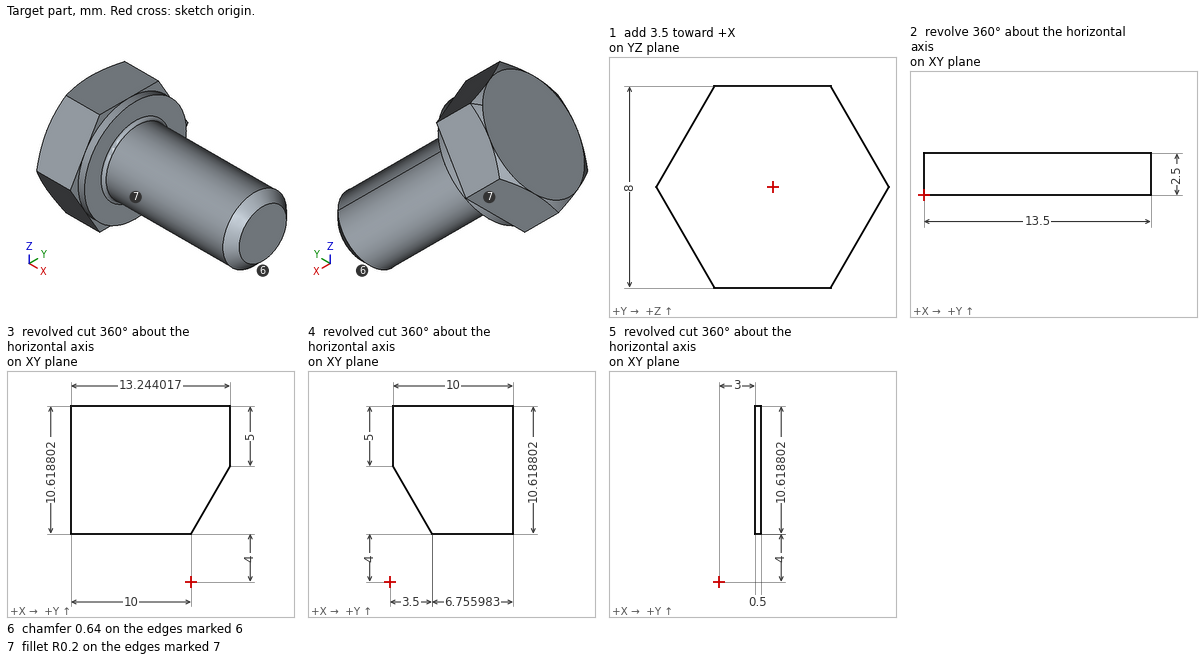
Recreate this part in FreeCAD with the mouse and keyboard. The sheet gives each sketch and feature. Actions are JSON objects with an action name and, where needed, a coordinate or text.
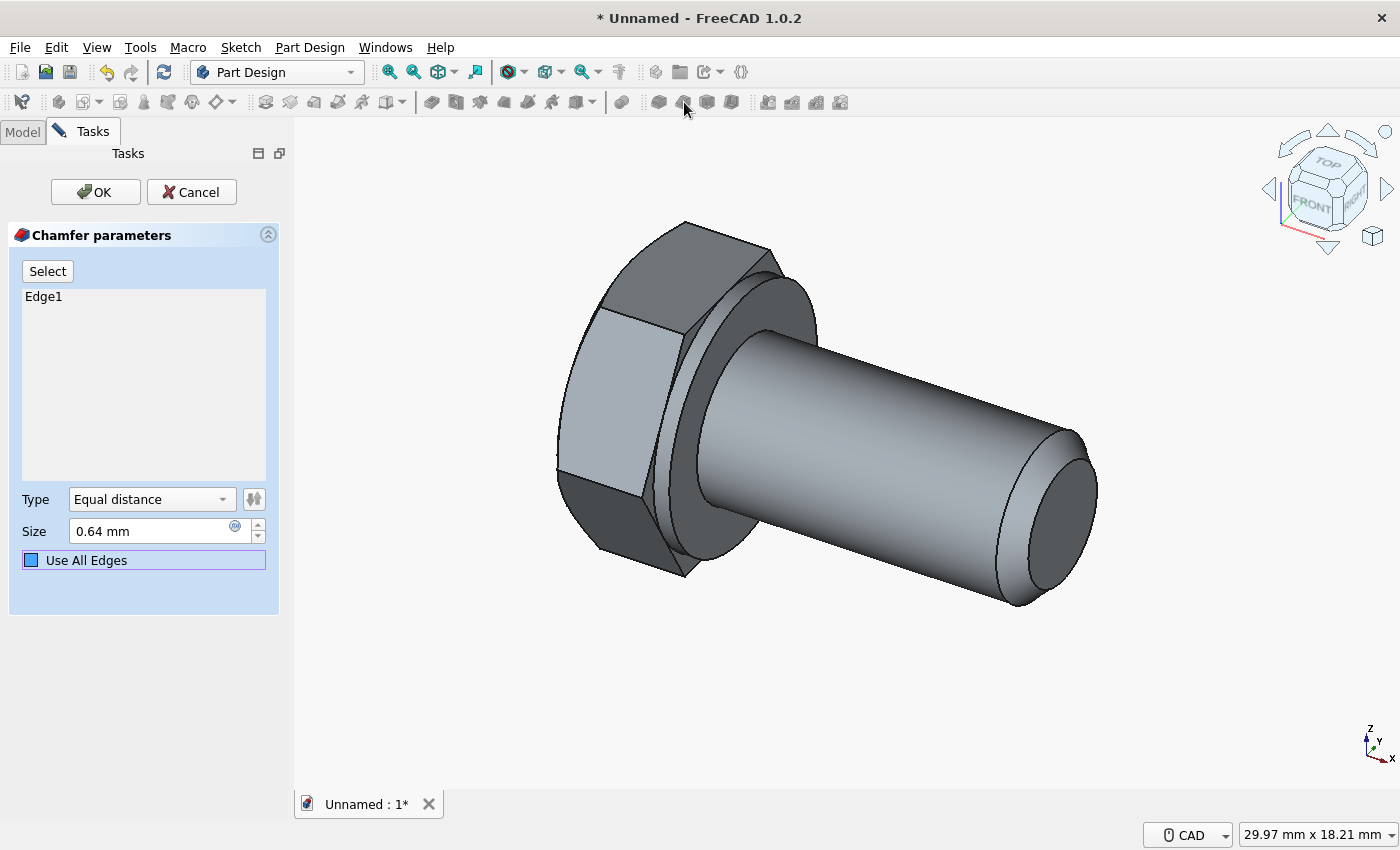
{"action": "left_click", "coordinate": [96, 192]}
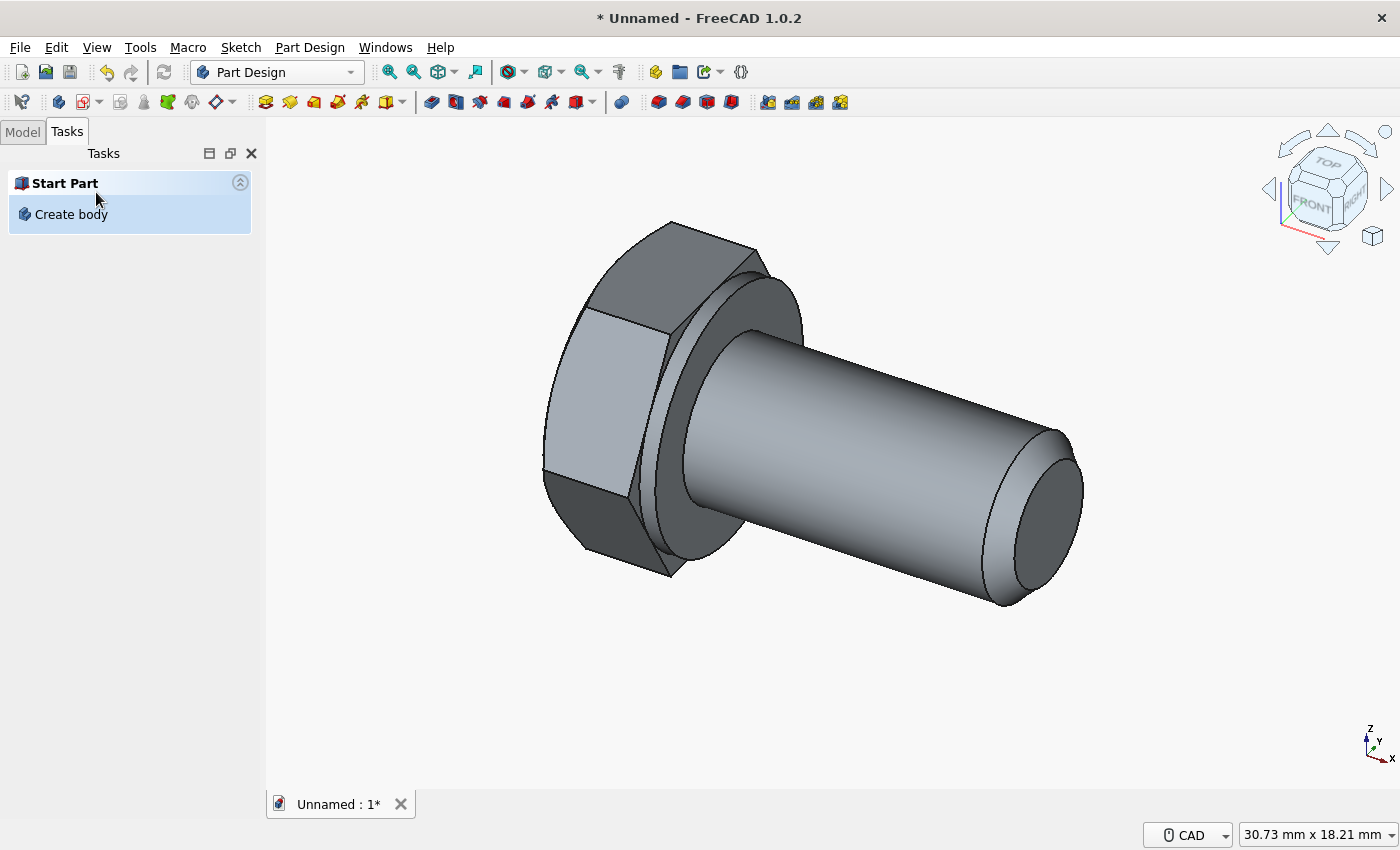
{"action": "key", "text": "0"}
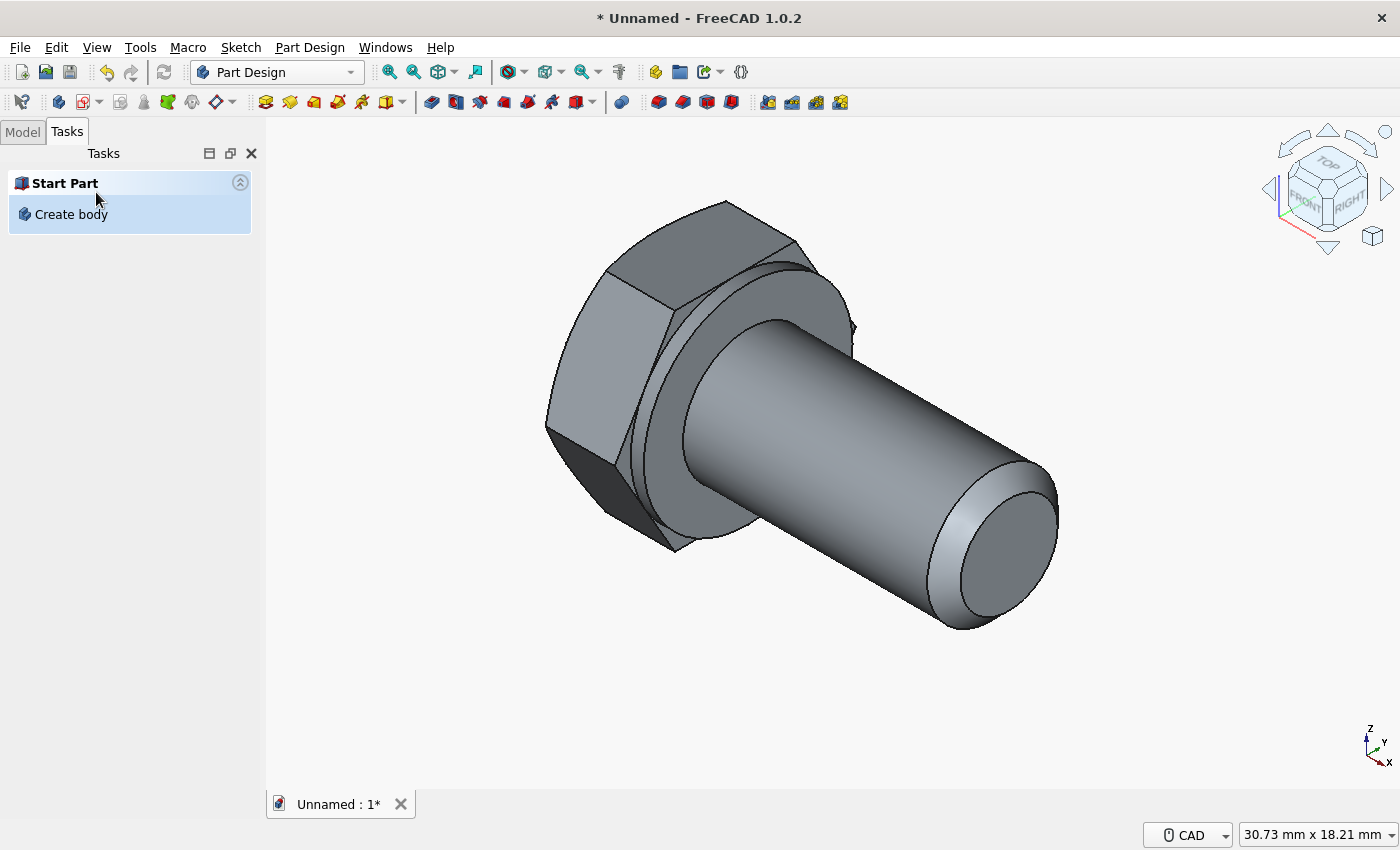
{"action": "key", "text": "2"}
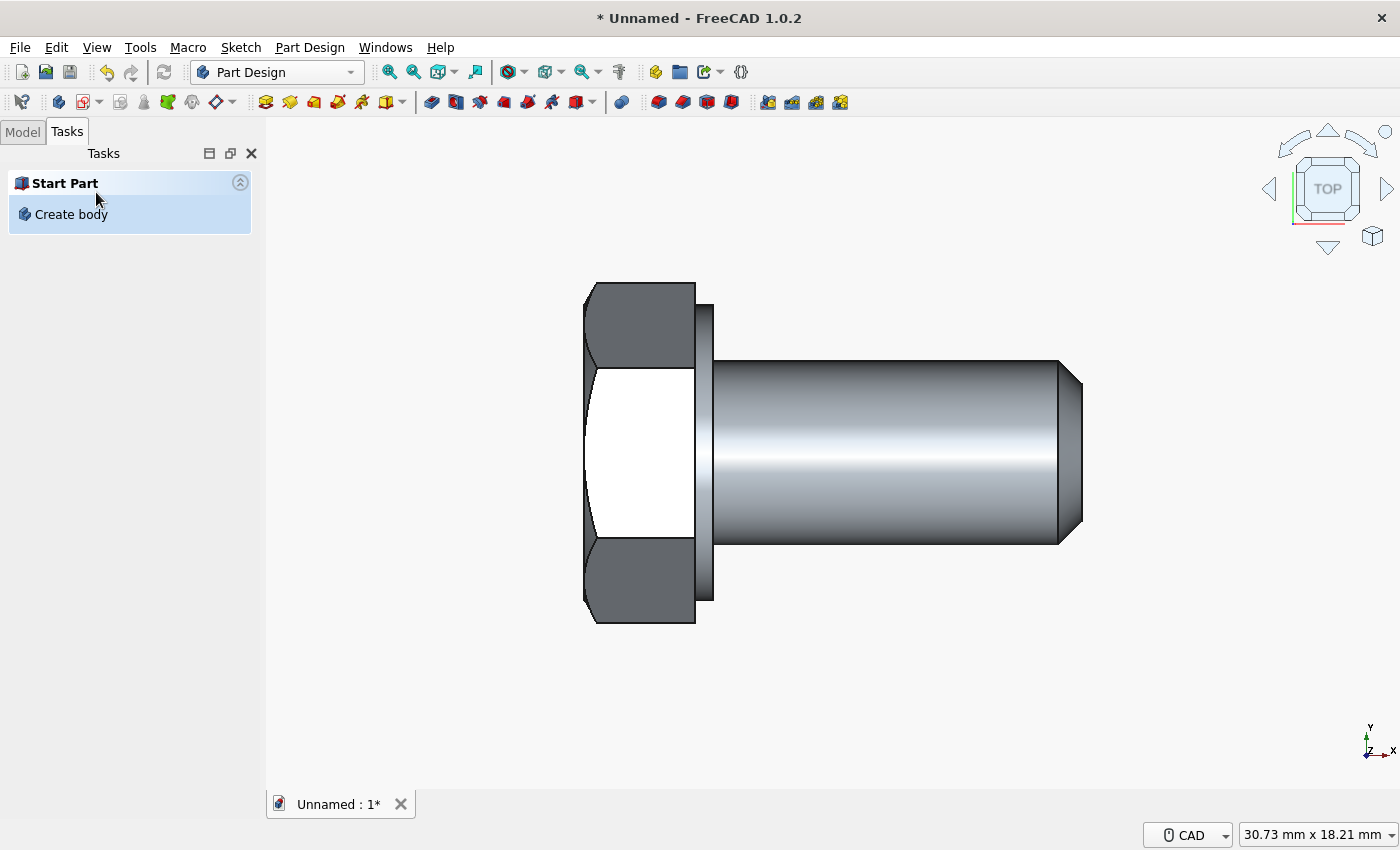
{"action": "key", "text": "1"}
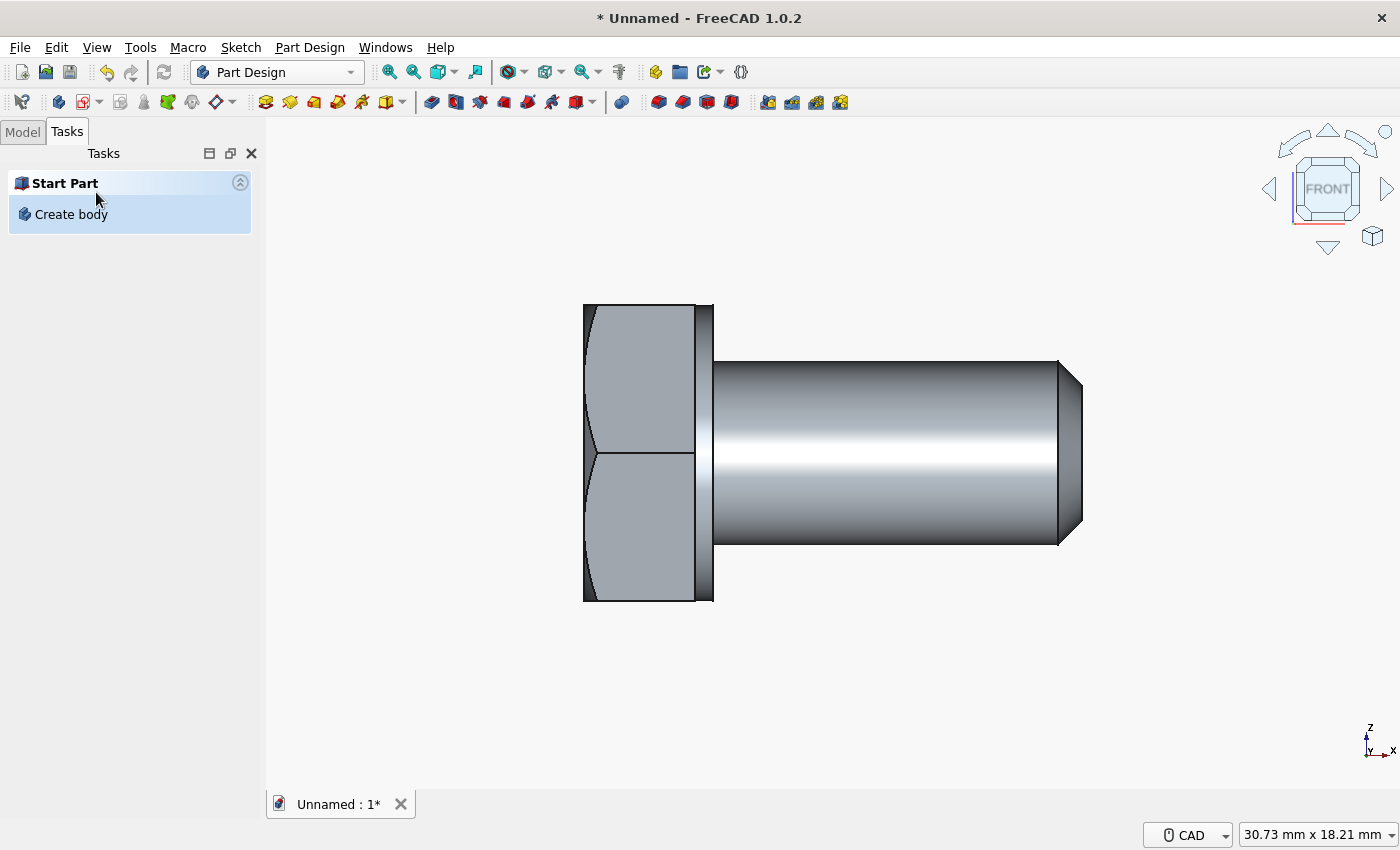
{"action": "left_click", "coordinate": [390, 72]}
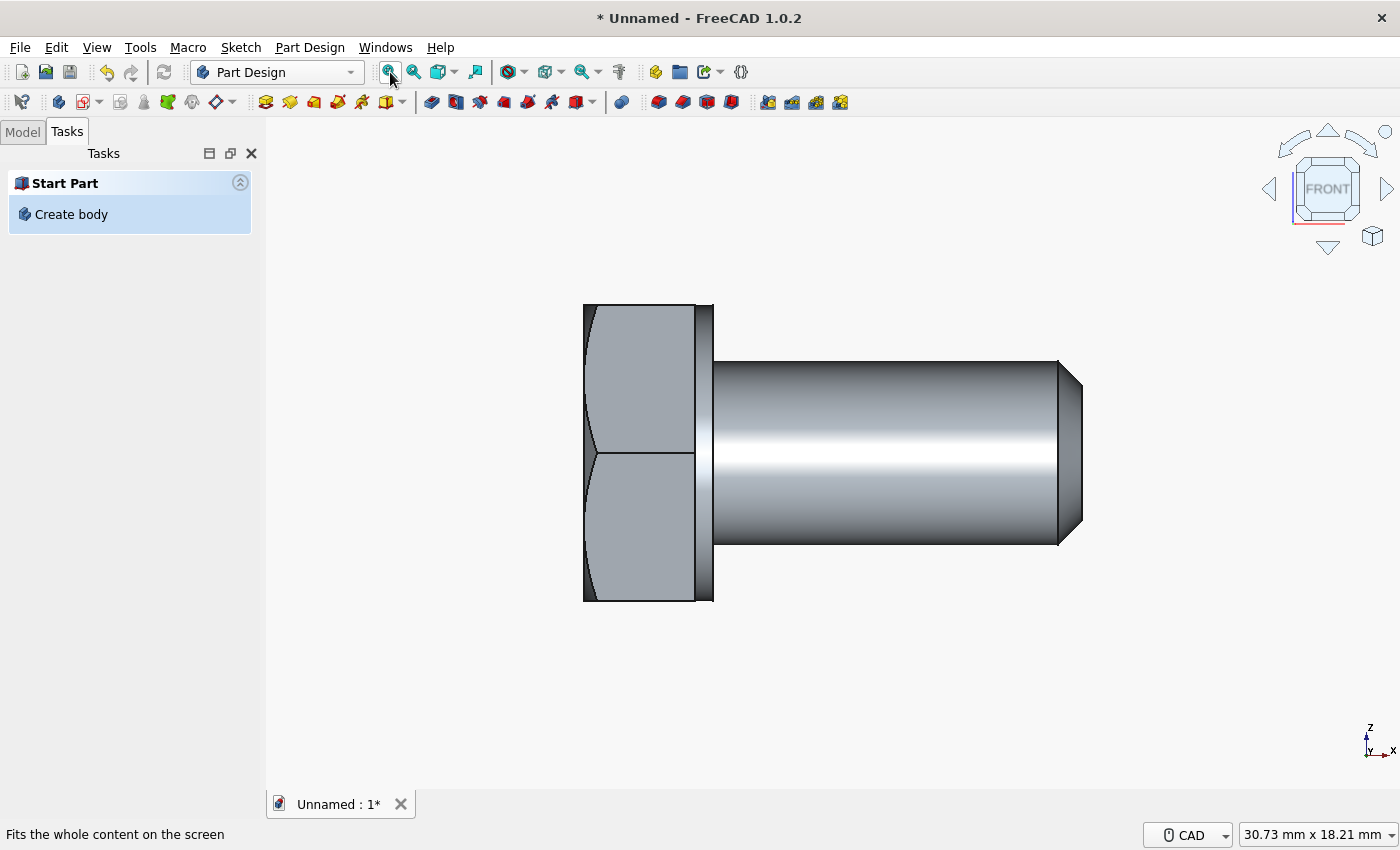
{"action": "key", "text": "3"}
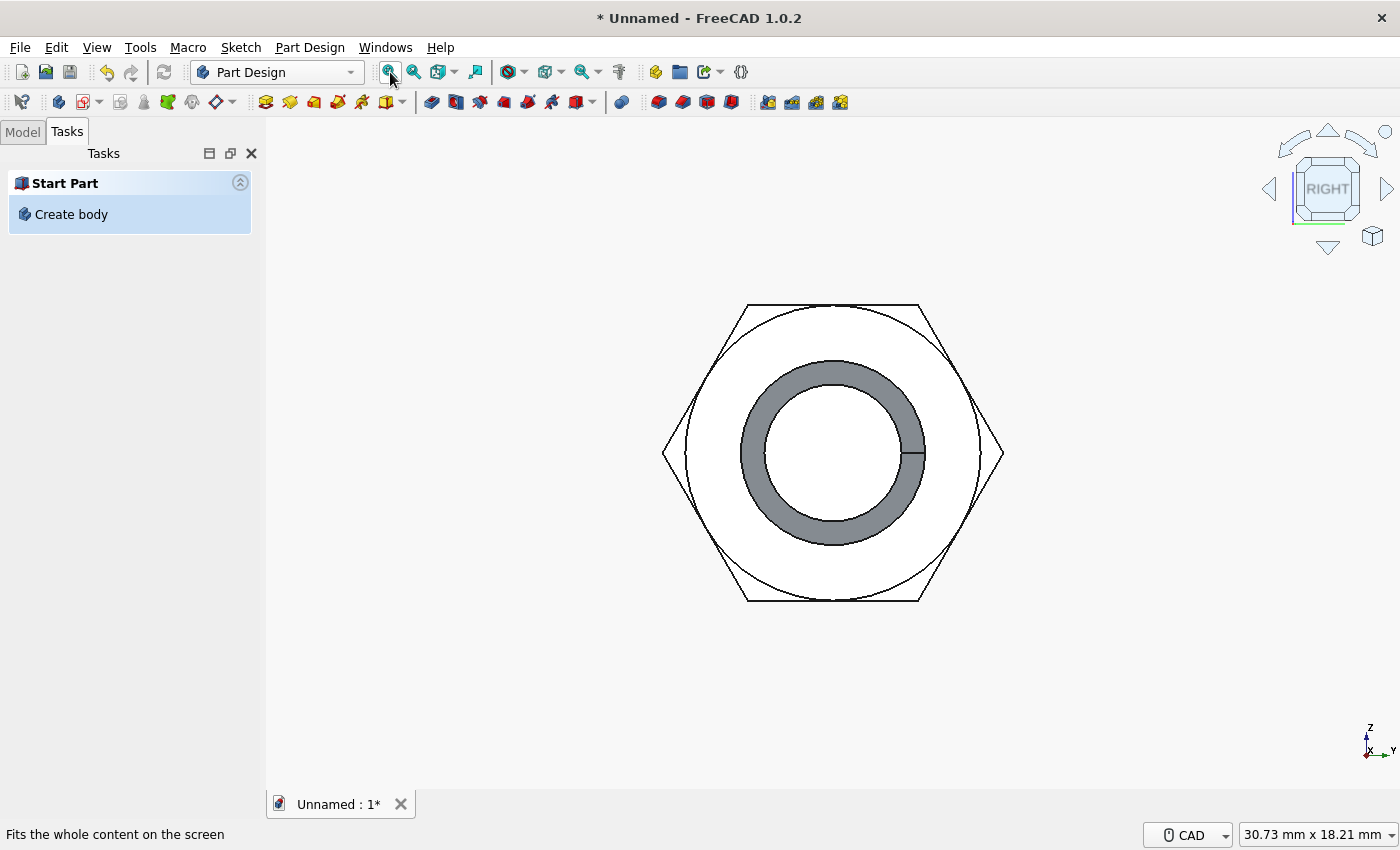
{"action": "left_click", "coordinate": [390, 72]}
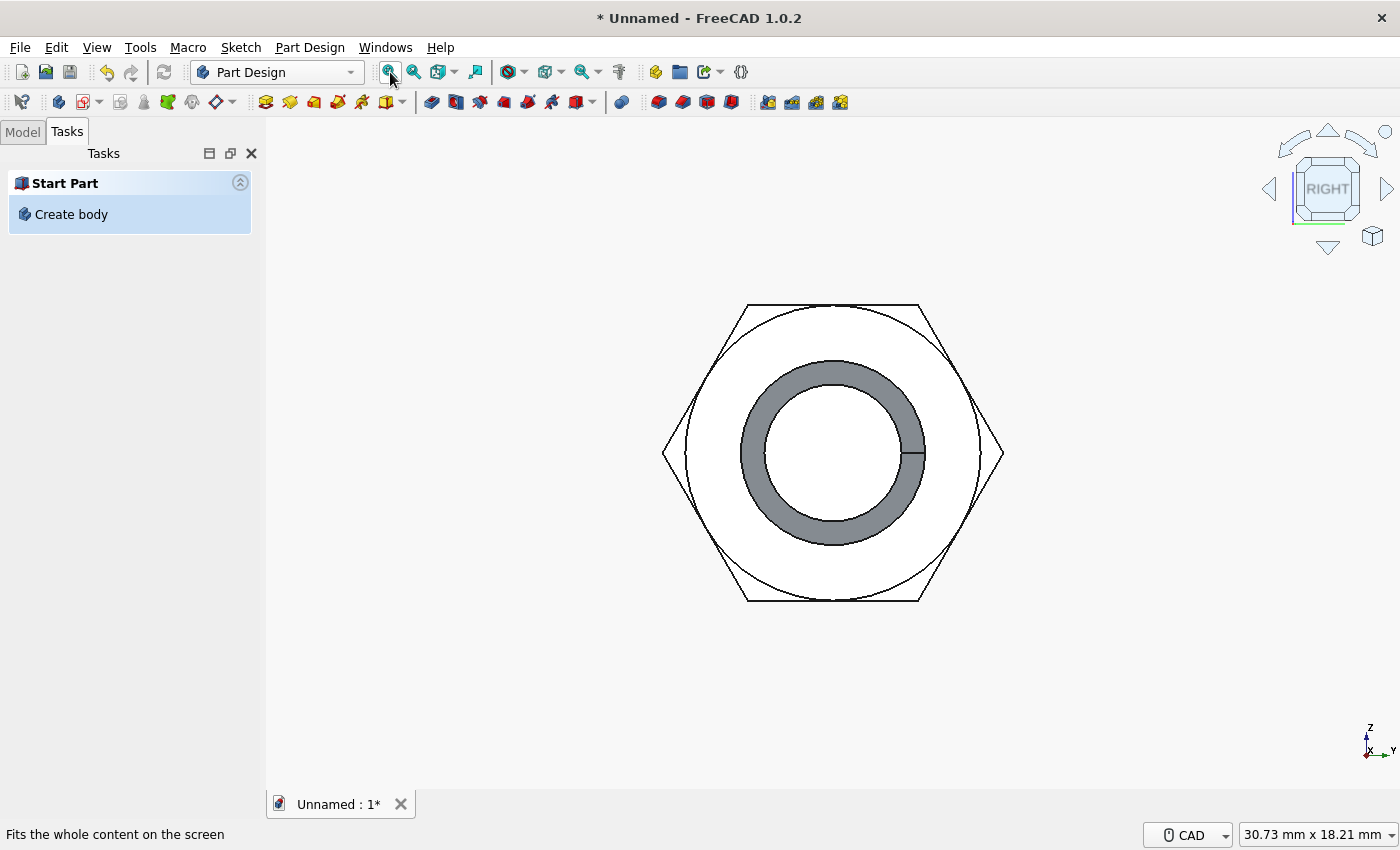
{"action": "key", "text": "5"}